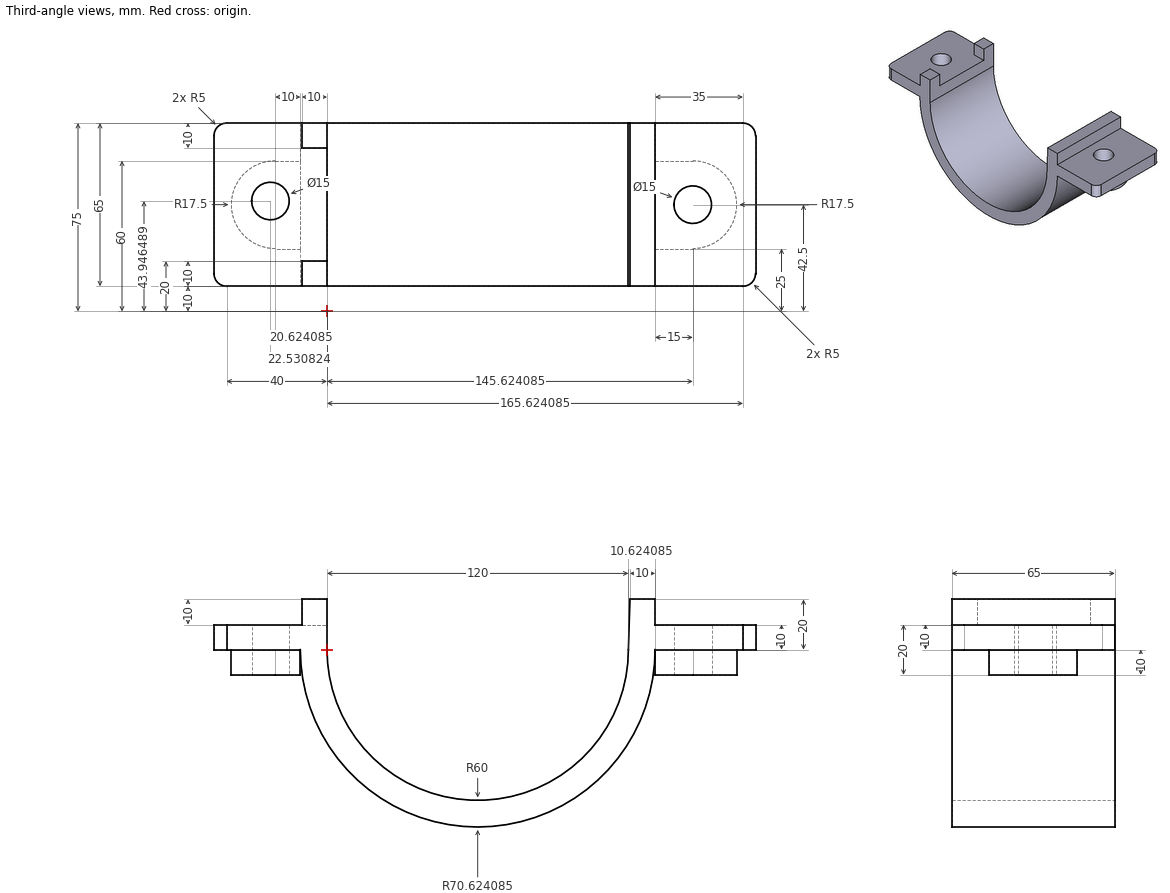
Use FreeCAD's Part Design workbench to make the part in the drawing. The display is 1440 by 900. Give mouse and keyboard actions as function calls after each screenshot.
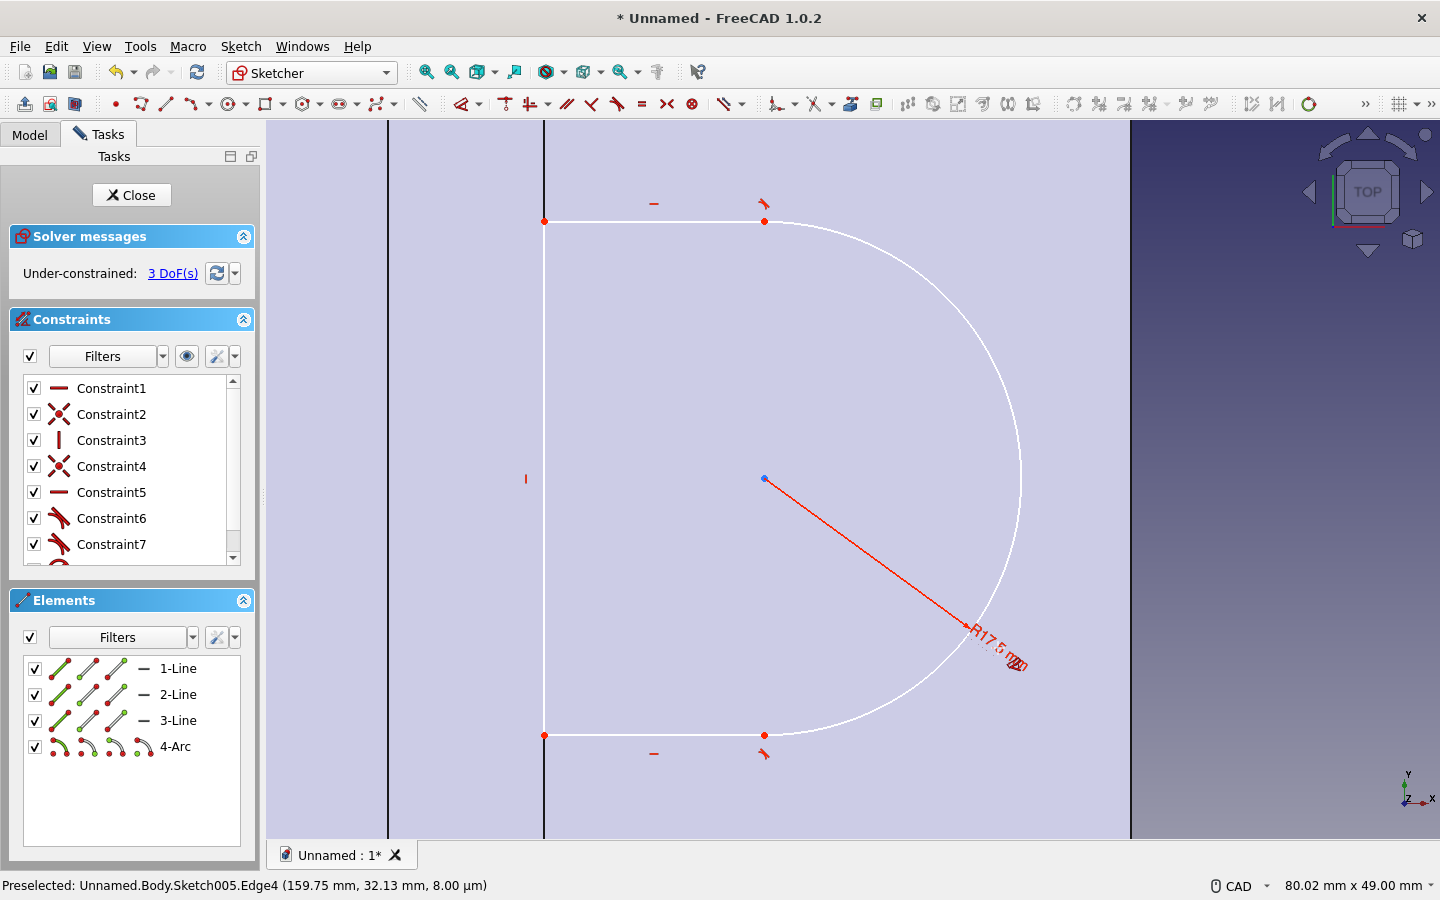
click(698, 735)
click(654, 769)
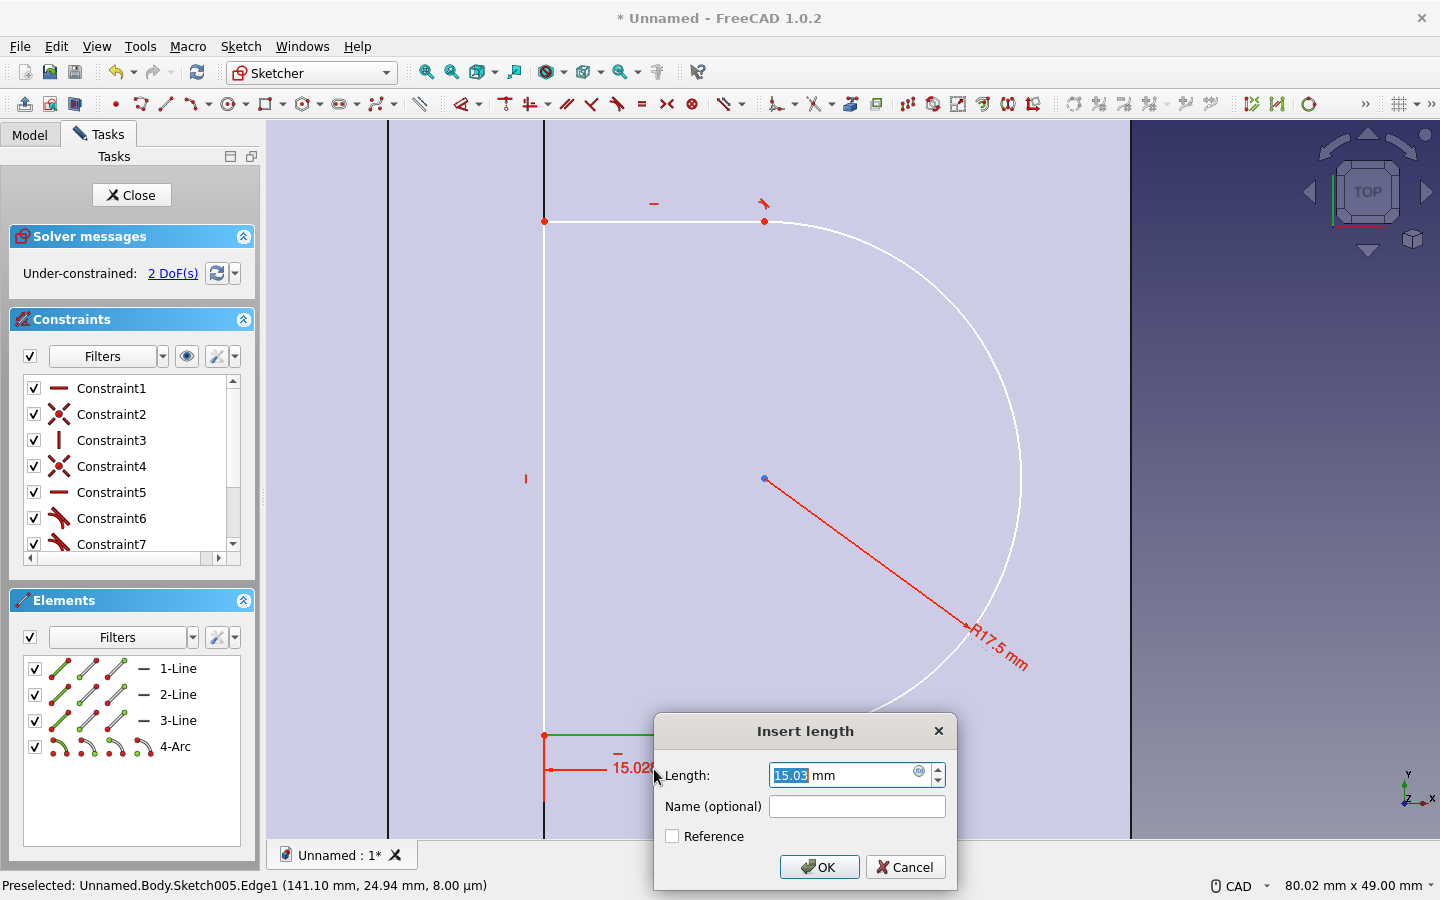
text(15)
key(Return)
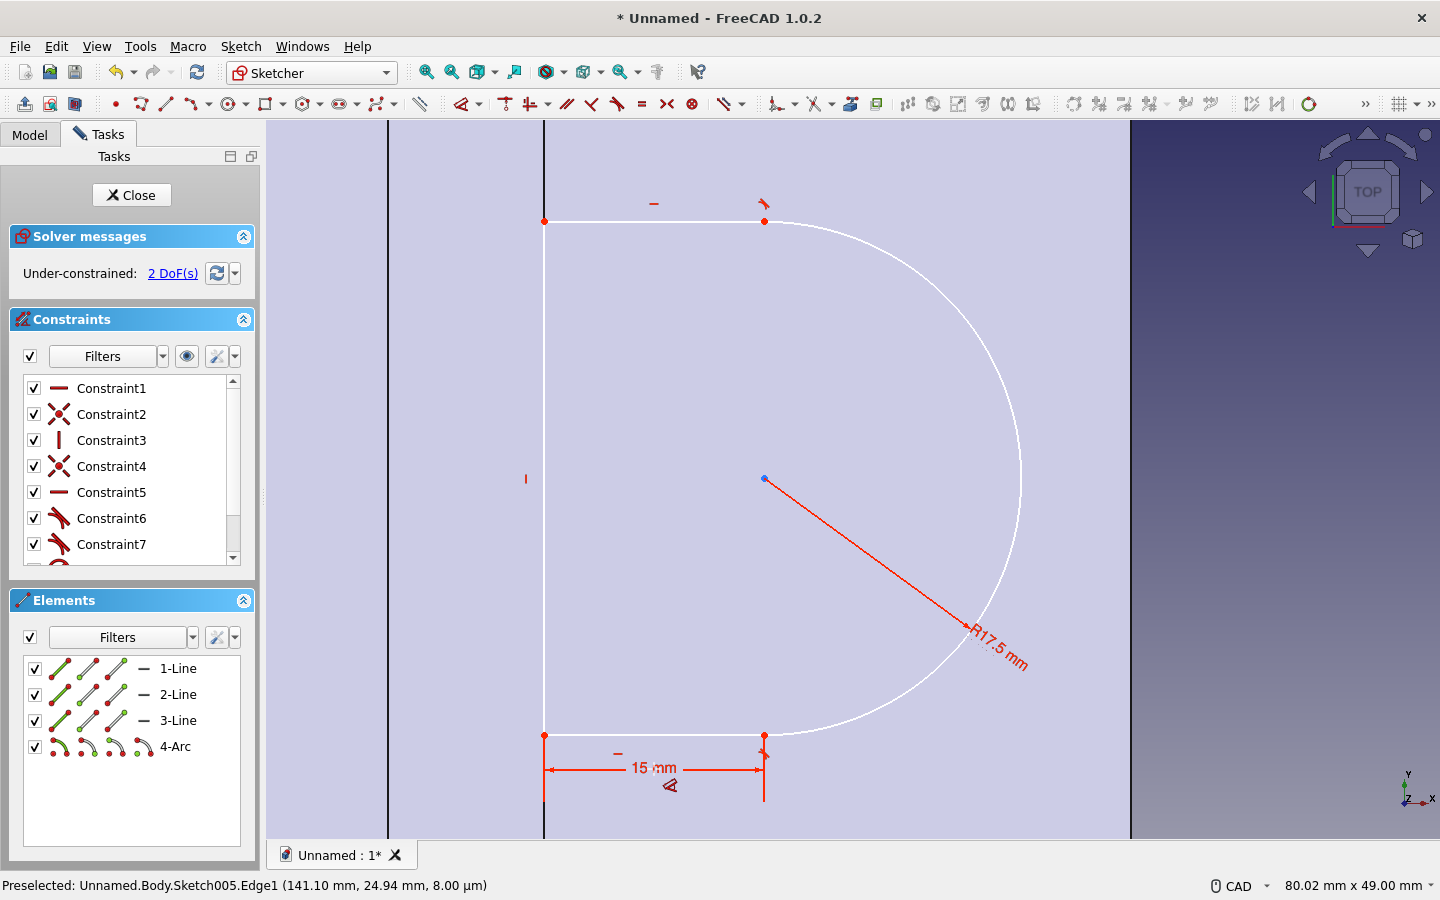
click(764, 735)
click(798, 773)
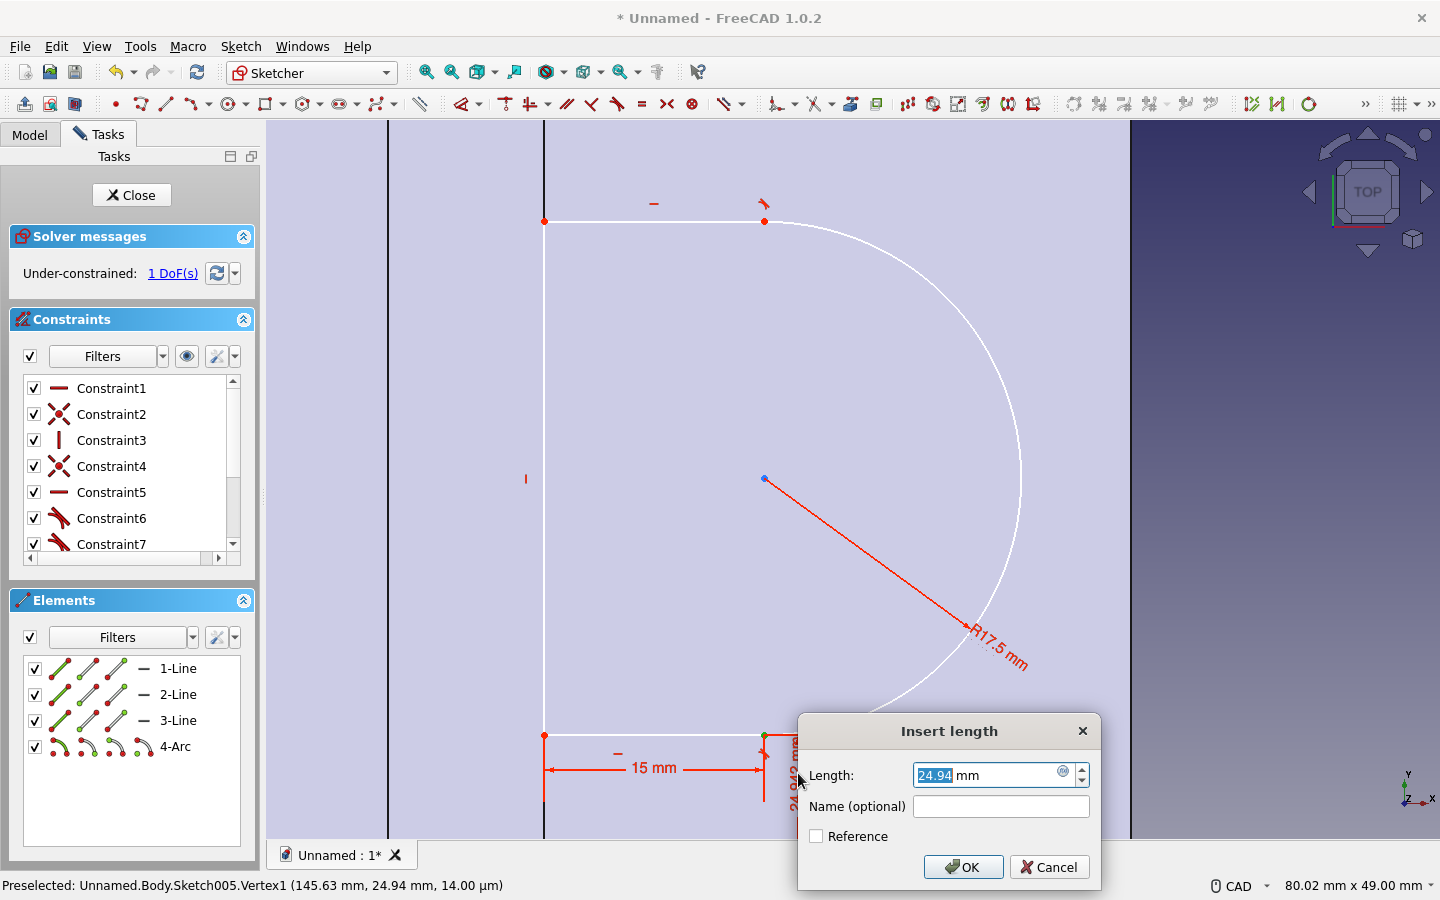
text(25)
key(Return)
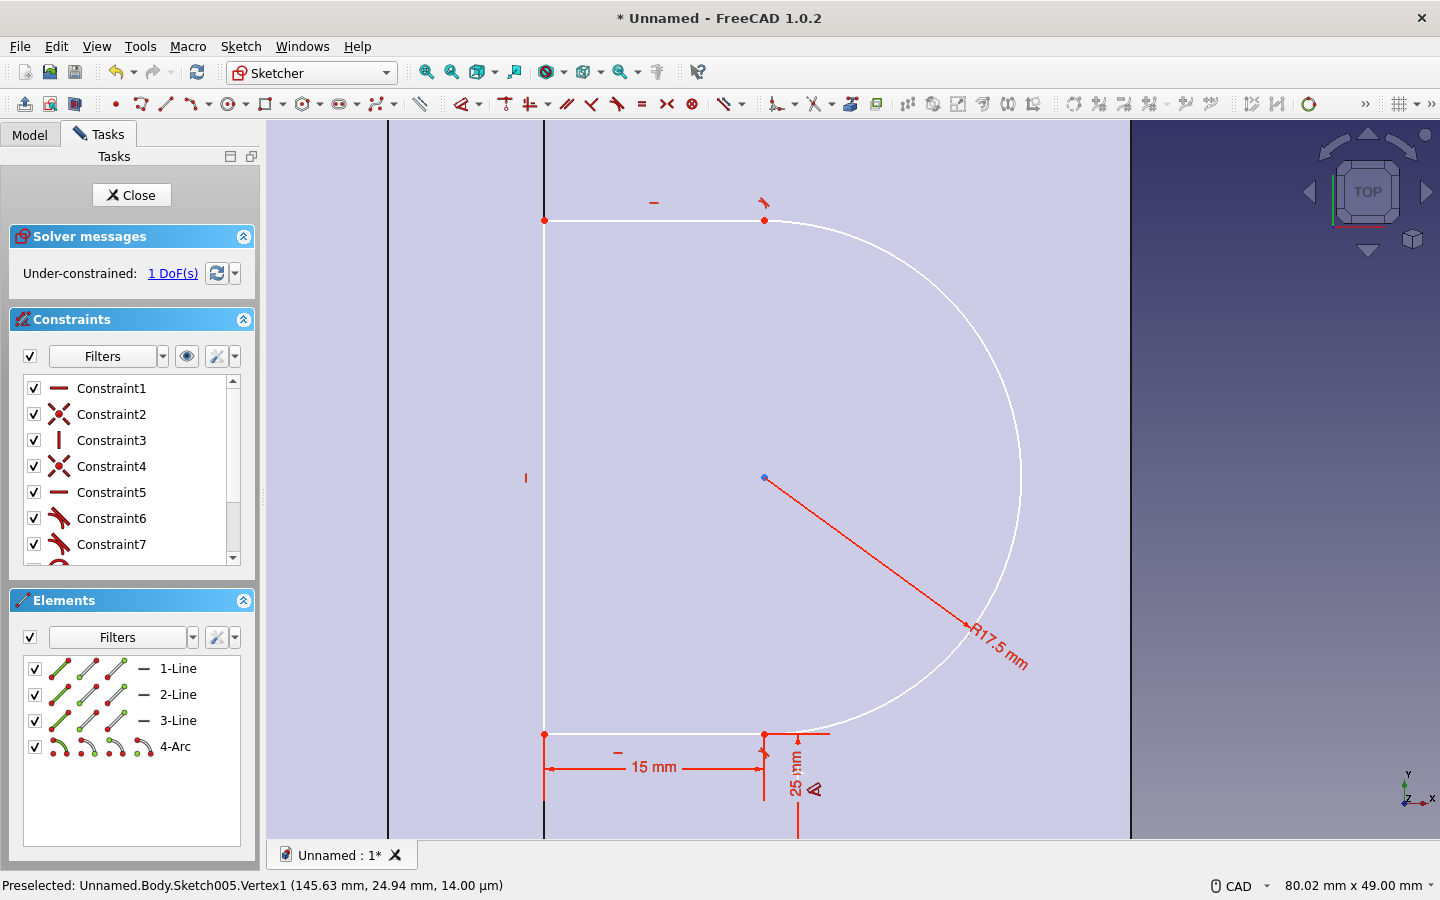
click(764, 734)
click(529, 700)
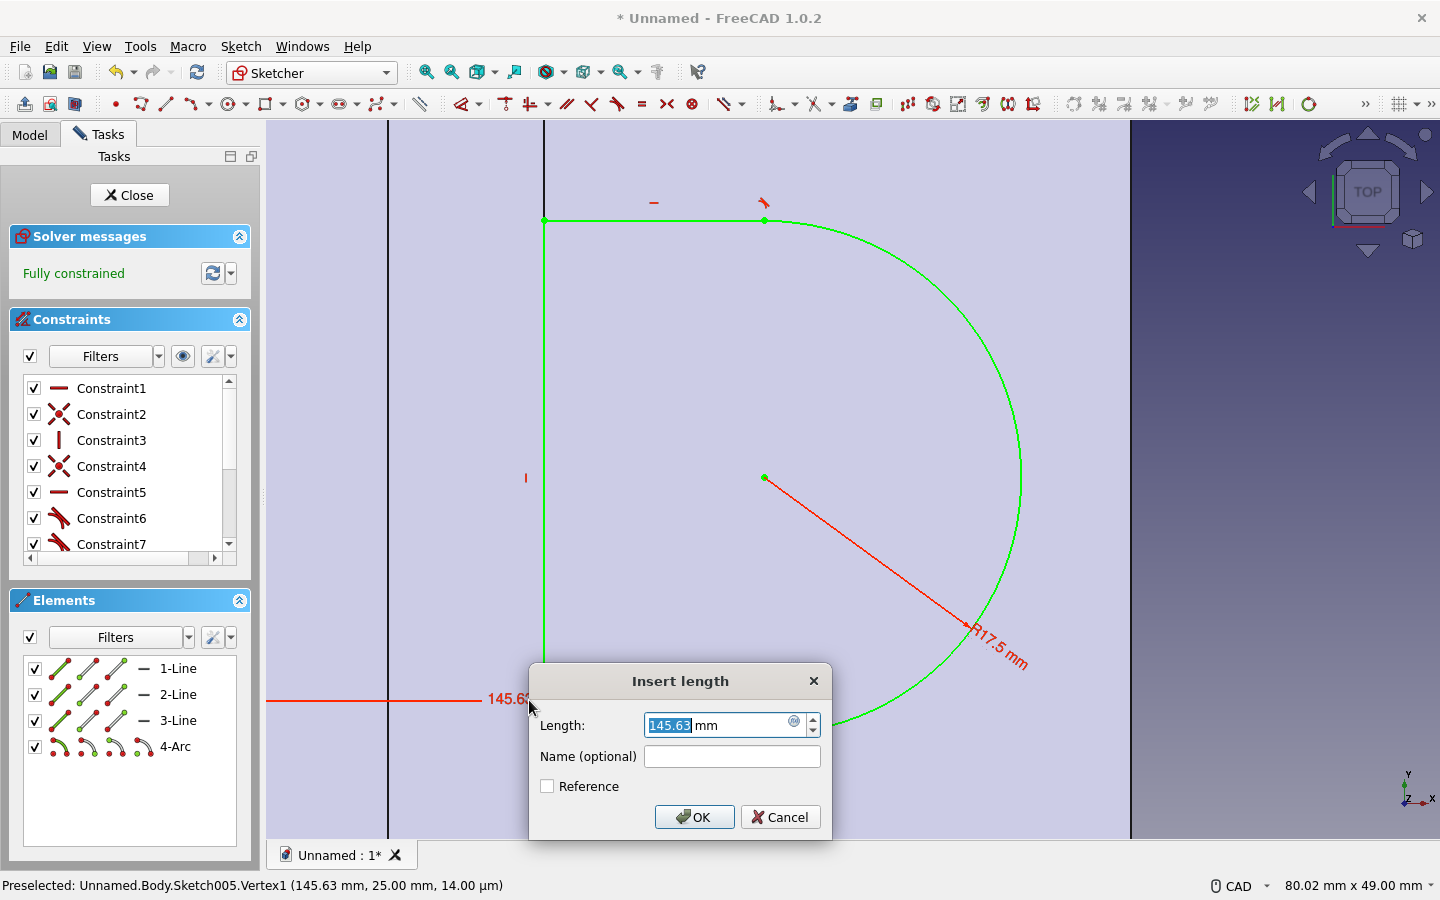
text(145.624085)
key(Return)
key(Escape)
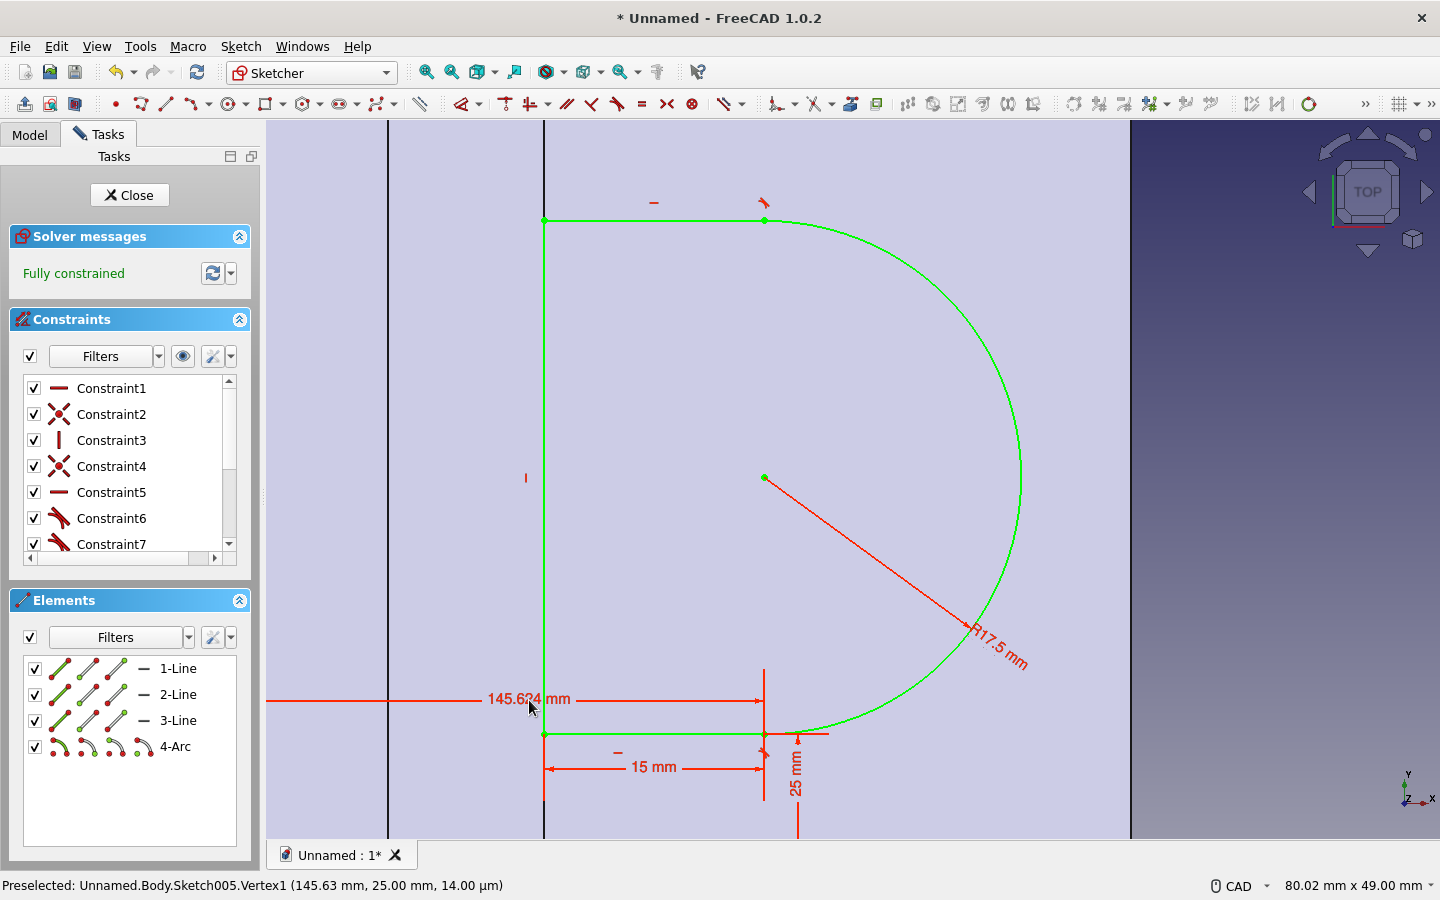
click(130, 195)